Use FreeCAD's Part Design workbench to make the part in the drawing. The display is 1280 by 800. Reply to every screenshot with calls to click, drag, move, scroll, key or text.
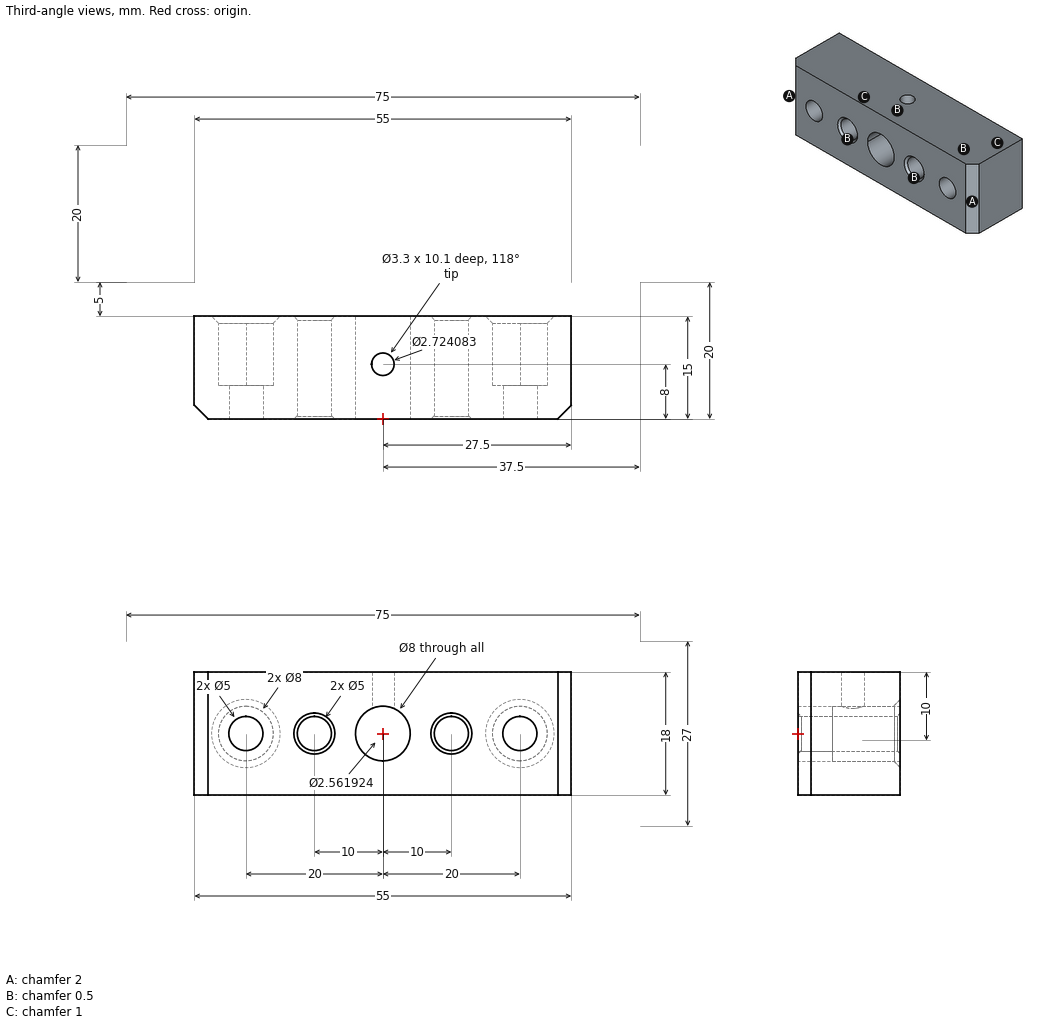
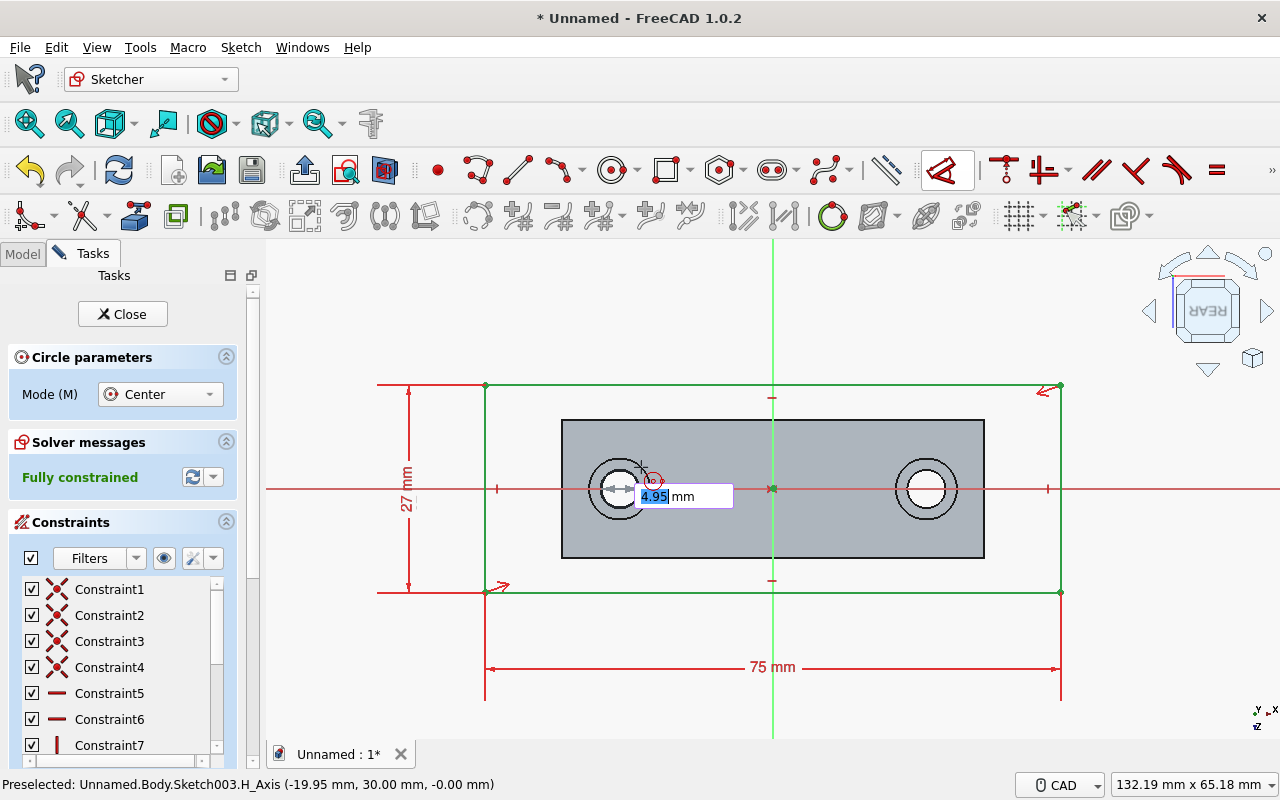
text(8)
key(Return)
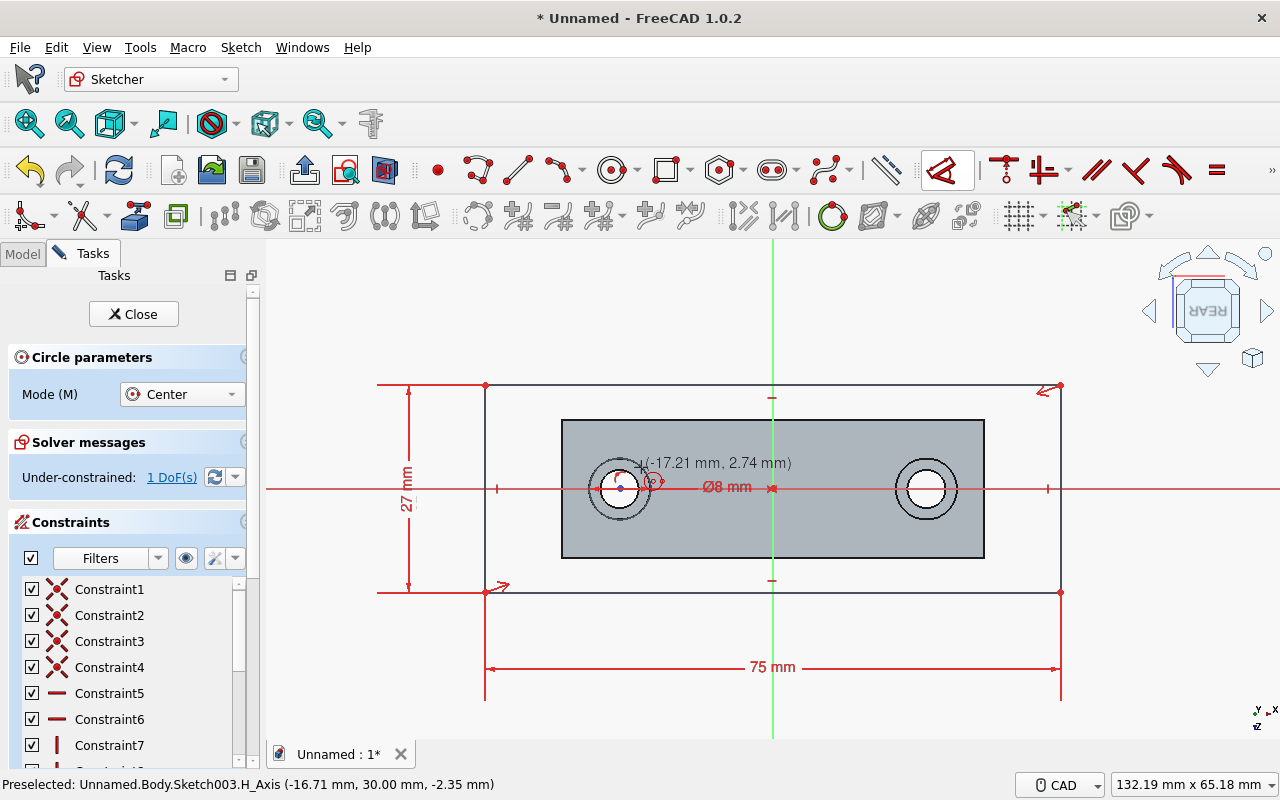
click(926, 489)
move(948, 467)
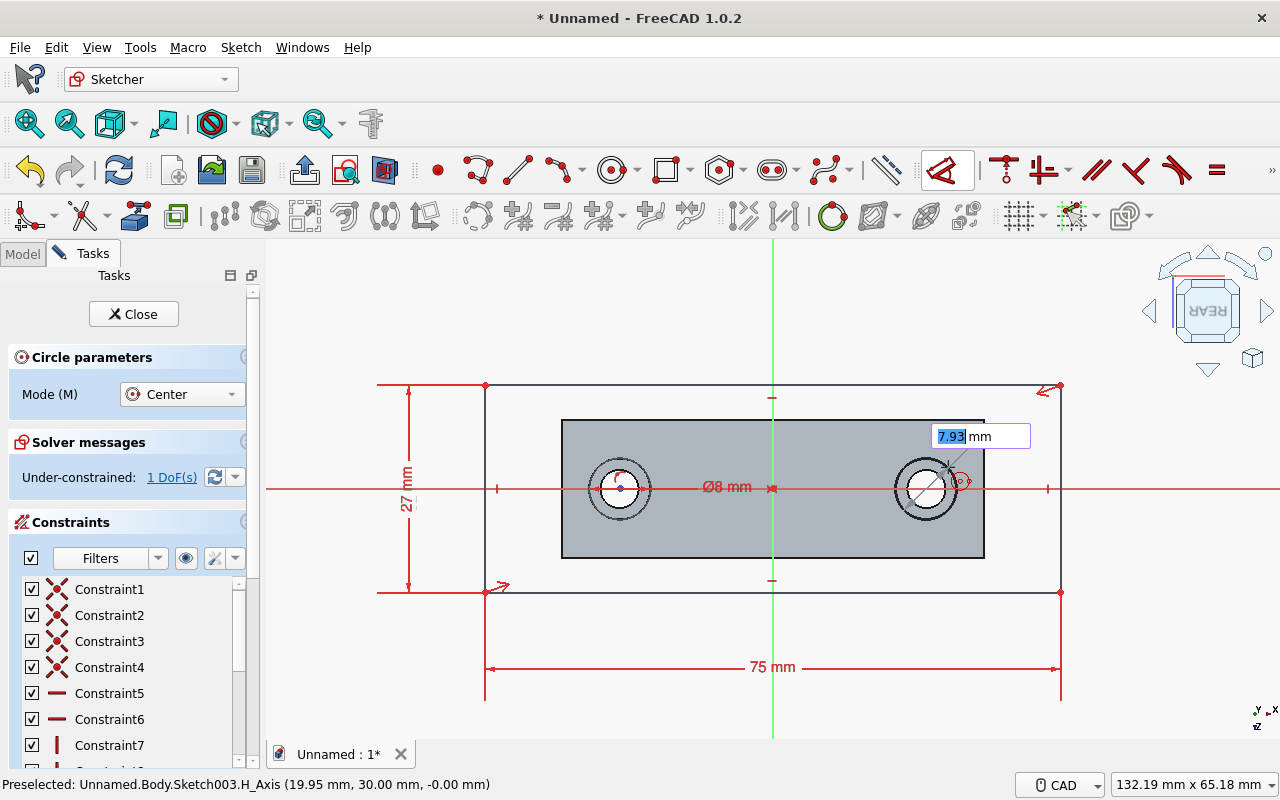
text(8)
key(Return)
key(Escape)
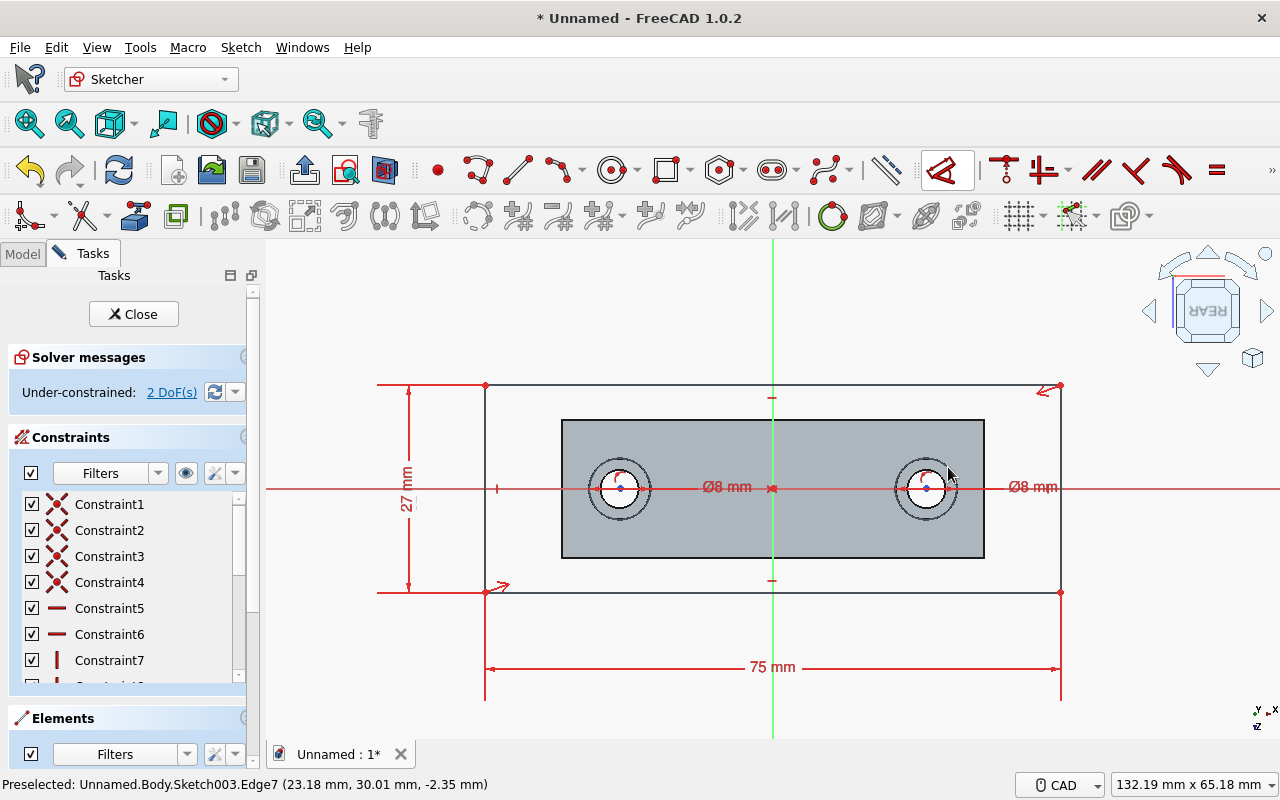
click(620, 489)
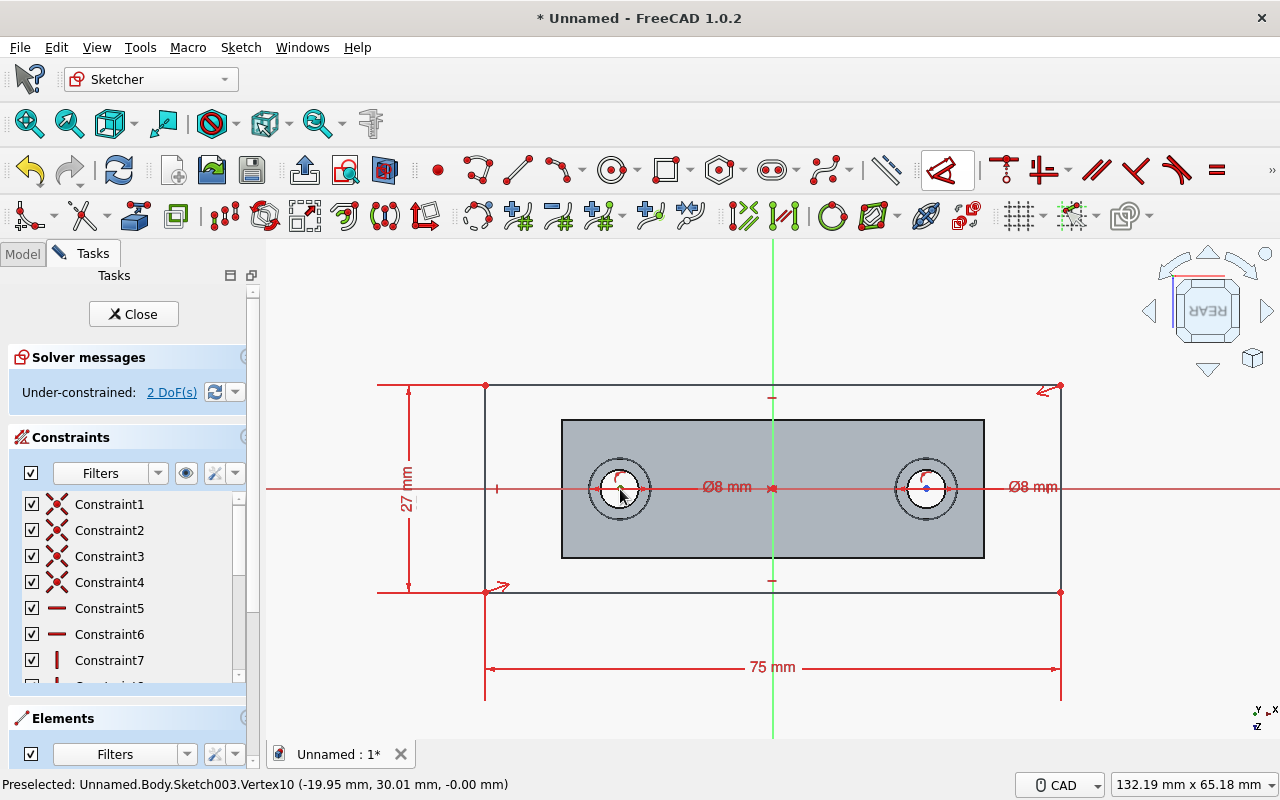
click(968, 170)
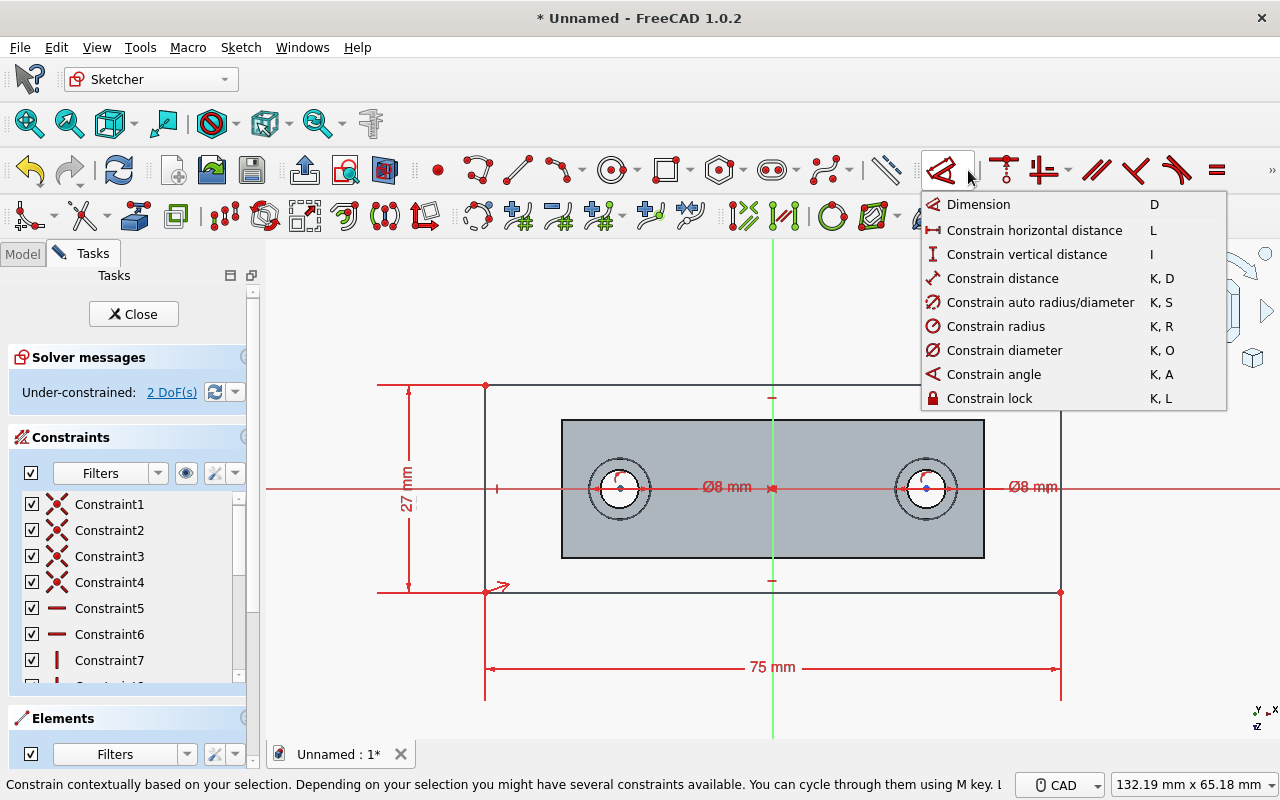
click(1074, 230)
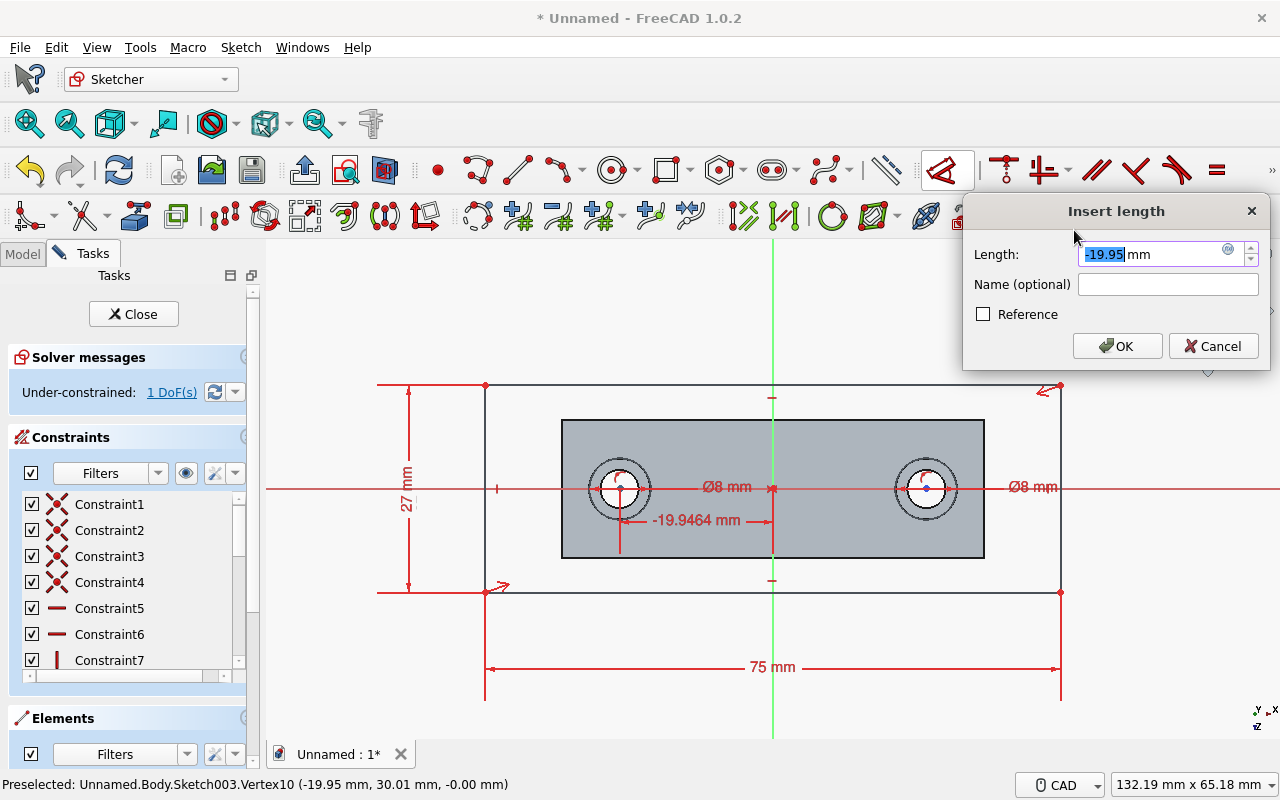
text(-20)
key(Return)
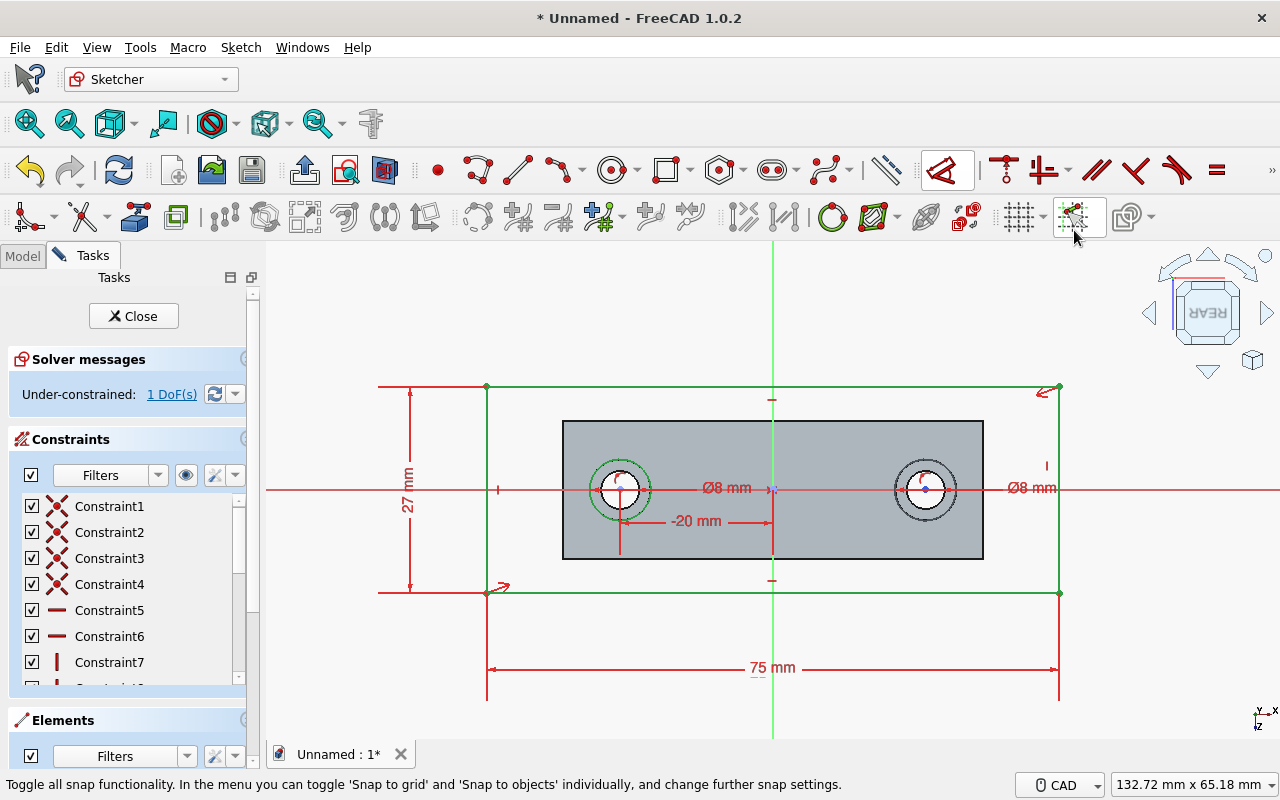
click(925, 490)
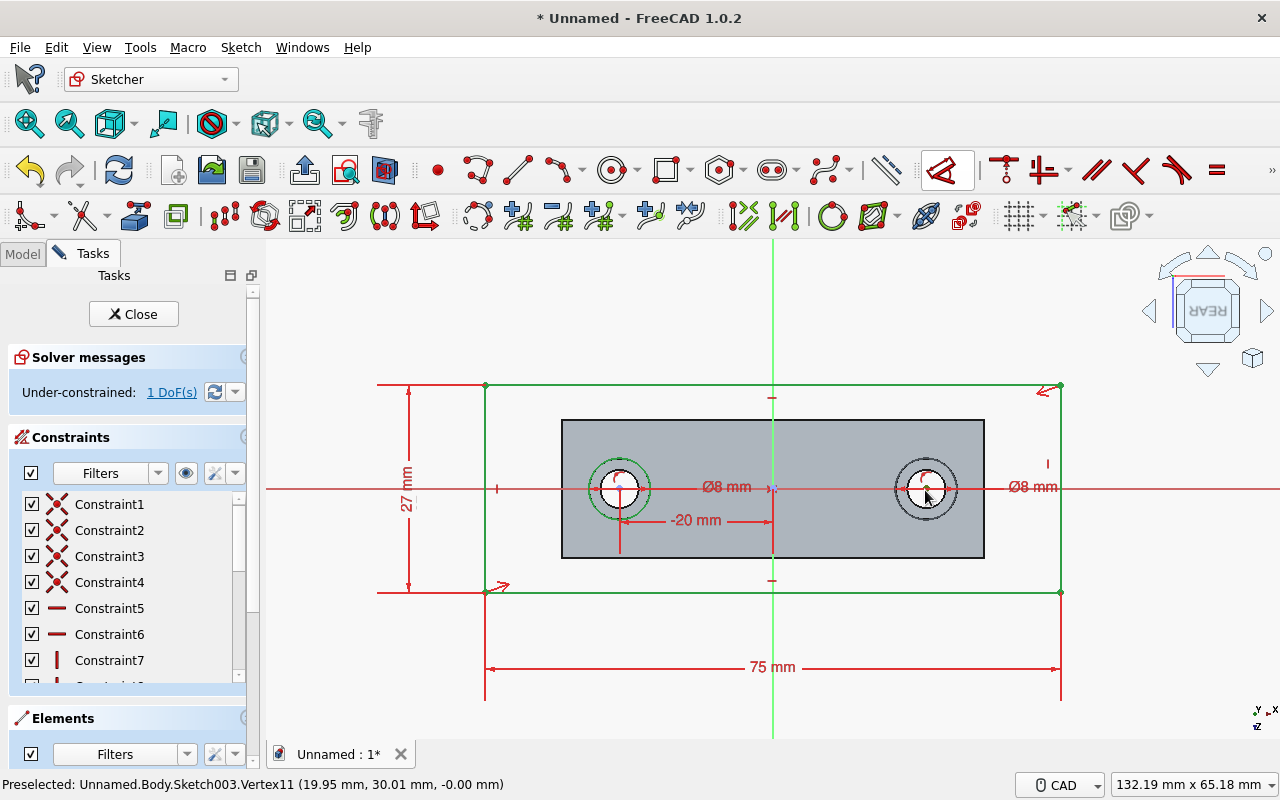
click(968, 170)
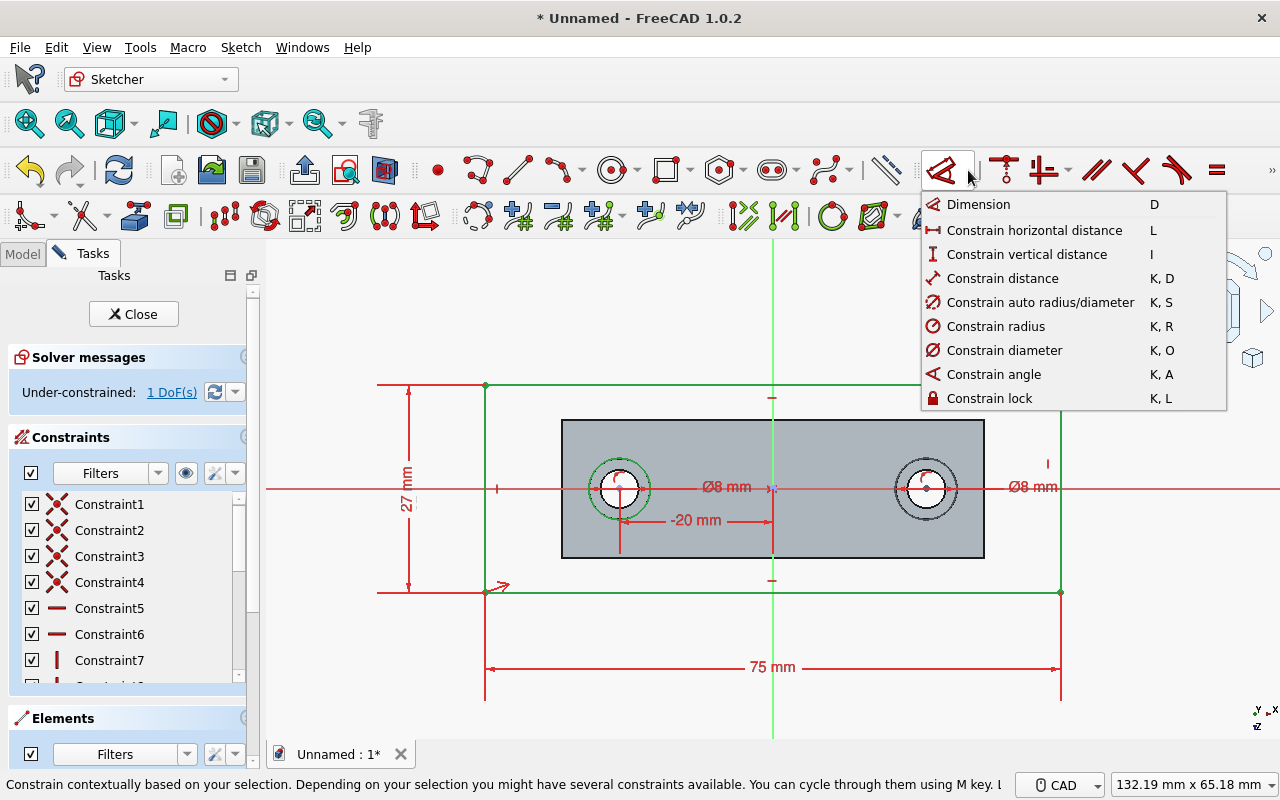
click(1074, 230)